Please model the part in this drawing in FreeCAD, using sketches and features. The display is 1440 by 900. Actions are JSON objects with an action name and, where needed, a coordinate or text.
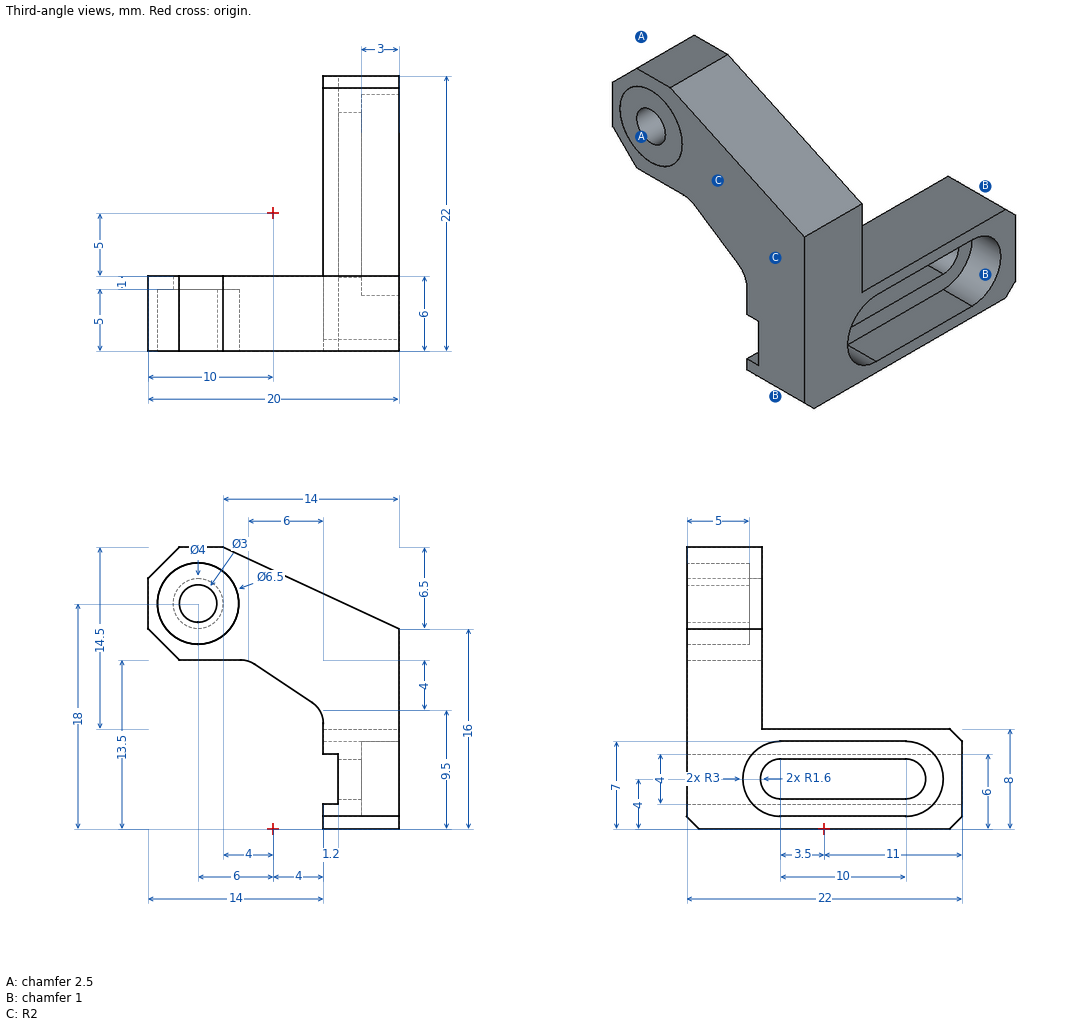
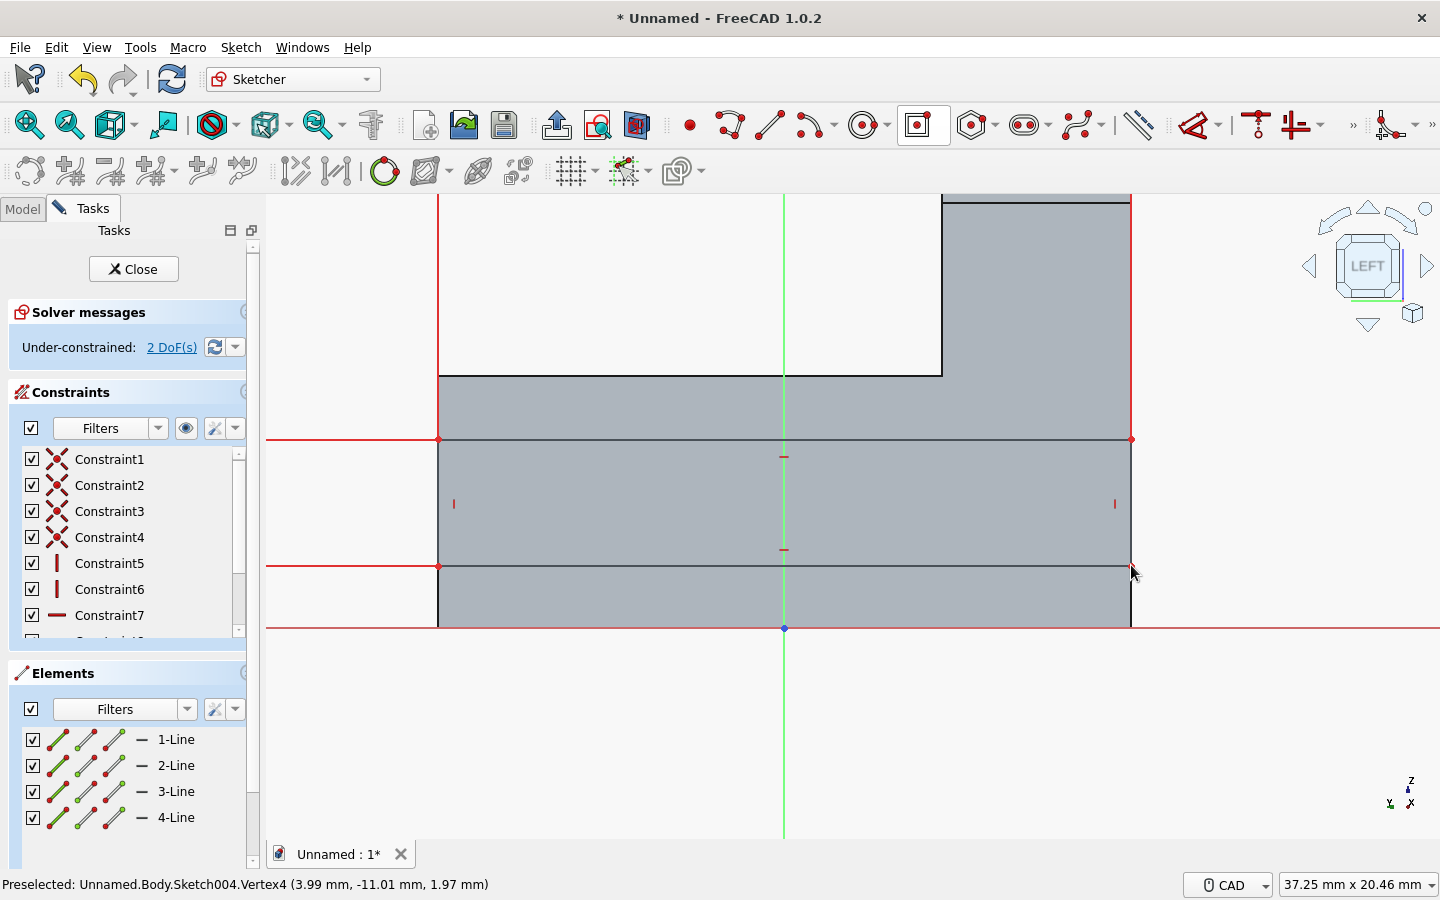
{"action": "left_click", "coordinate": [1194, 126]}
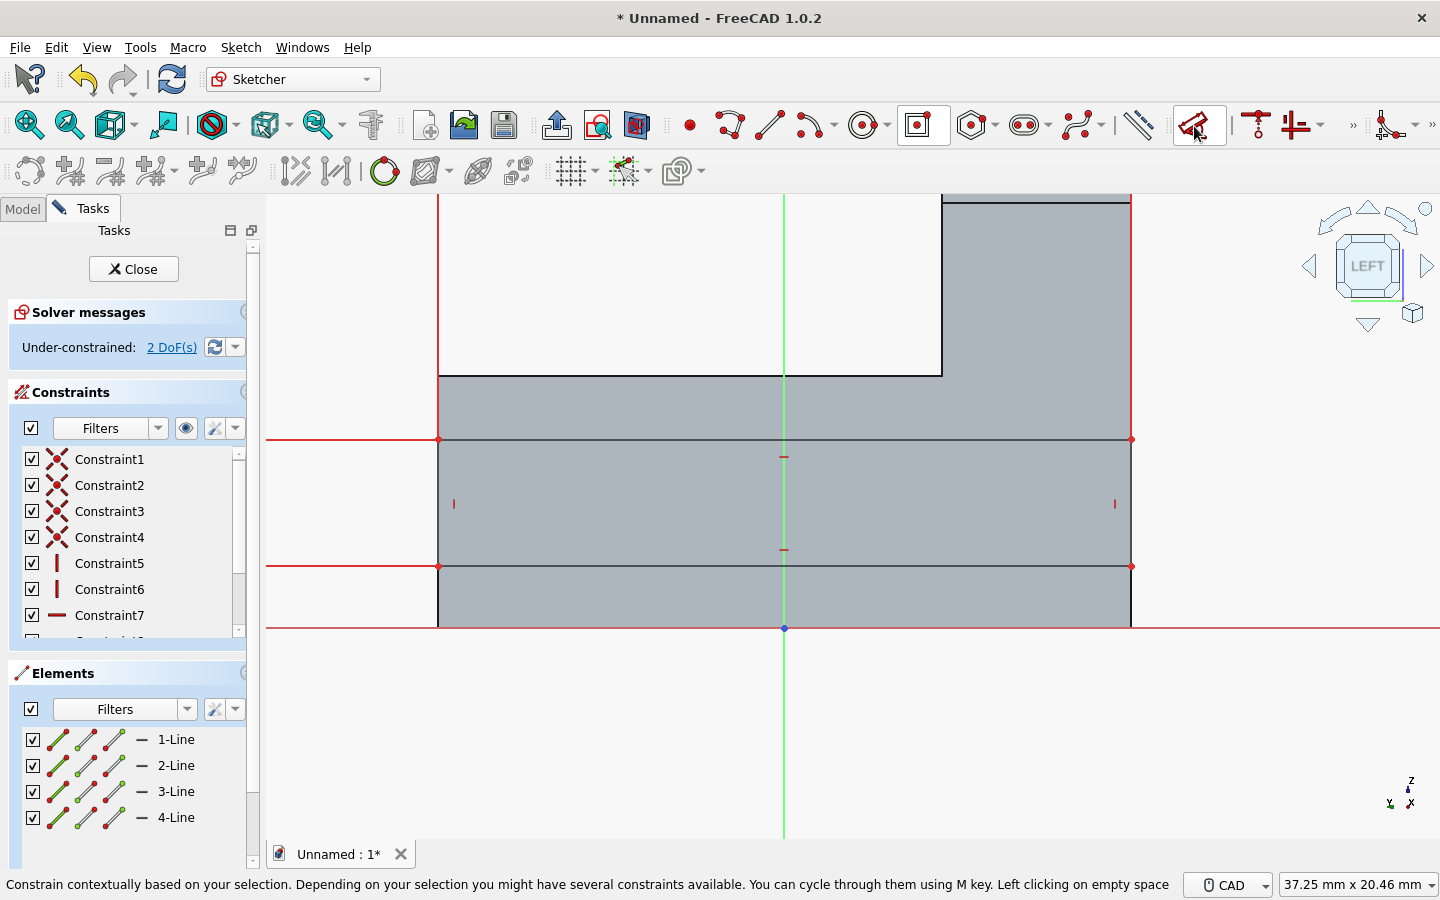
{"action": "left_click", "coordinate": [438, 440]}
{"action": "left_click", "coordinate": [404, 534]}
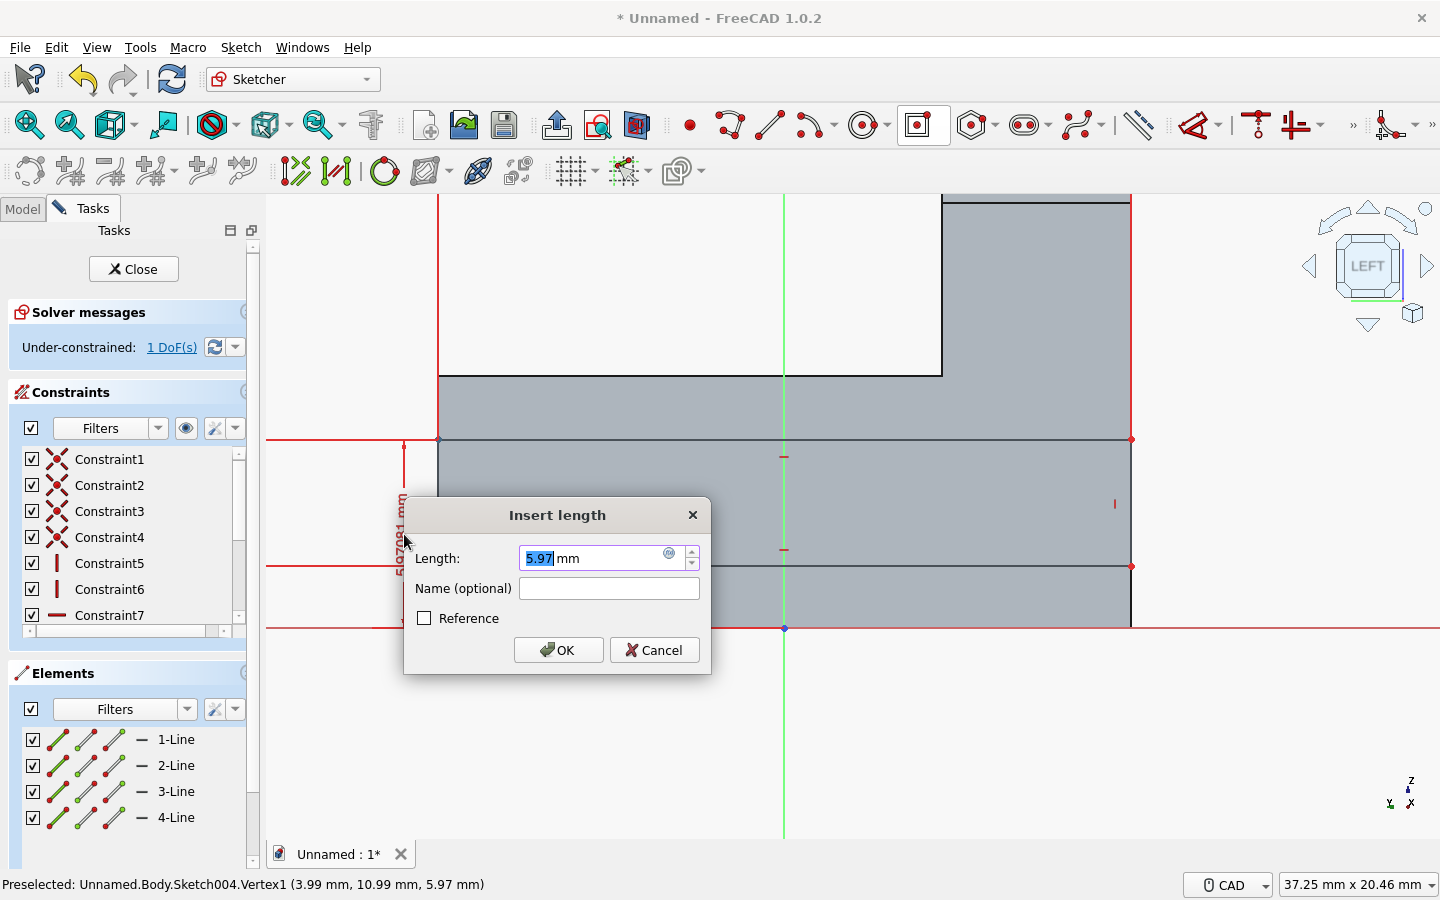
{"action": "type", "text": "6"}
{"action": "key", "text": "Return"}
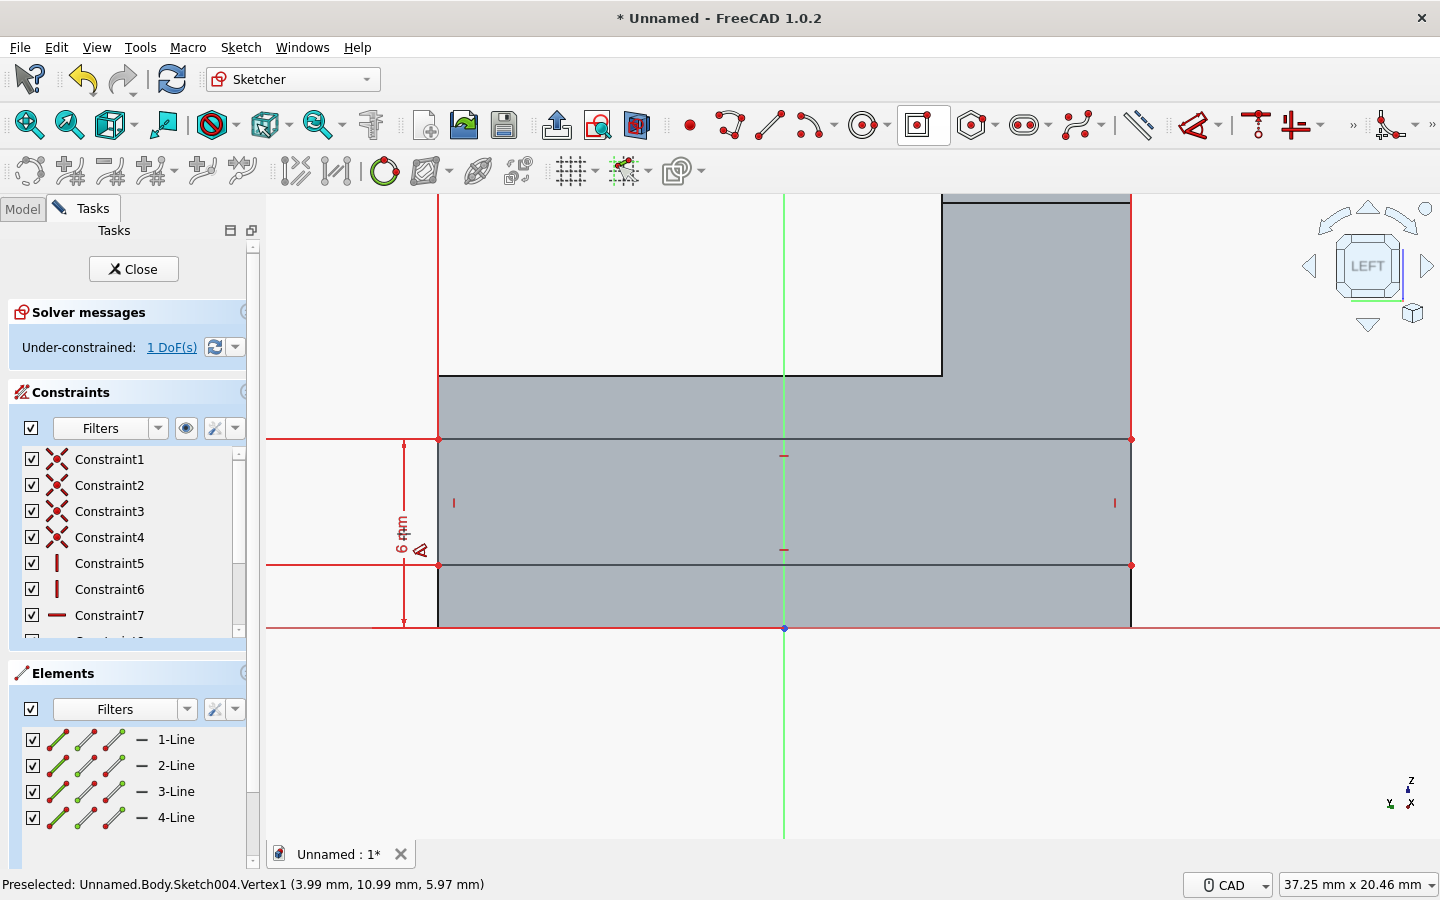
{"action": "left_click", "coordinate": [438, 439]}
{"action": "left_click", "coordinate": [611, 662]}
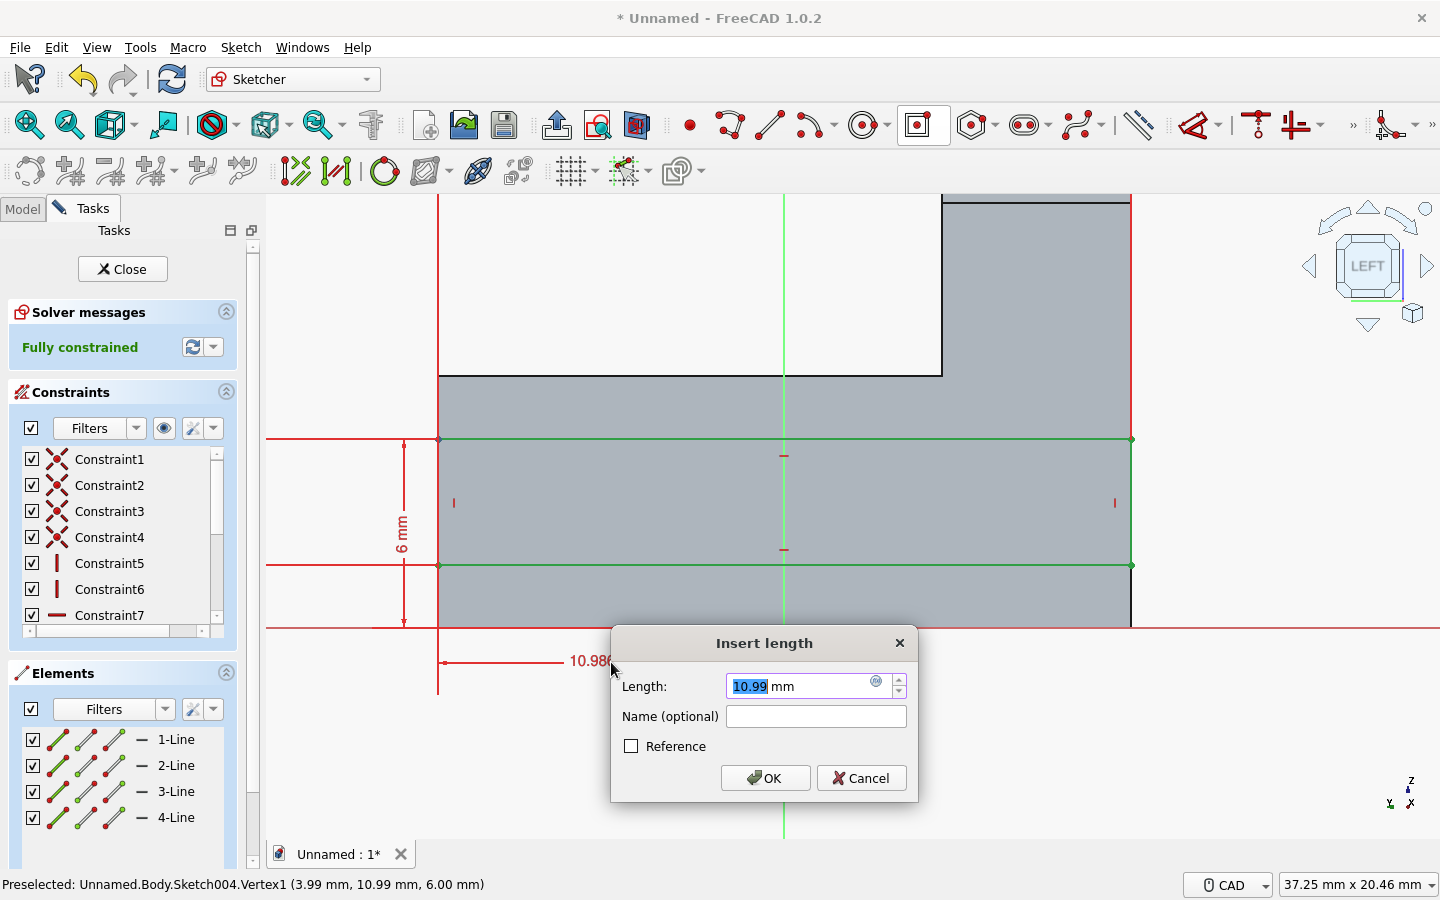
{"action": "type", "text": "11"}
{"action": "key", "text": "Return"}
{"action": "key", "text": "Escape"}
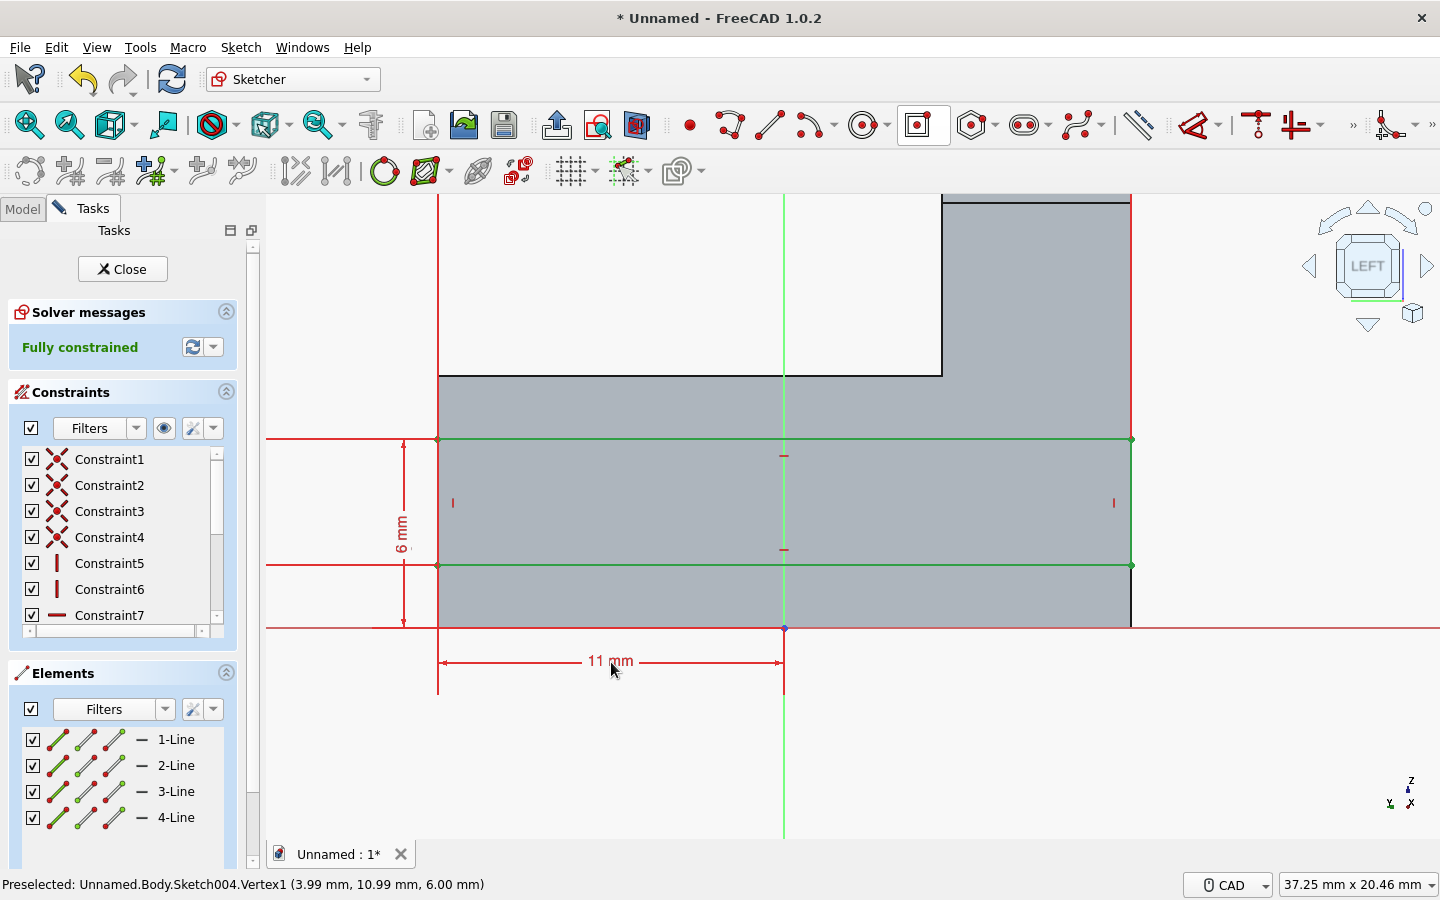
{"action": "left_click", "coordinate": [123, 269]}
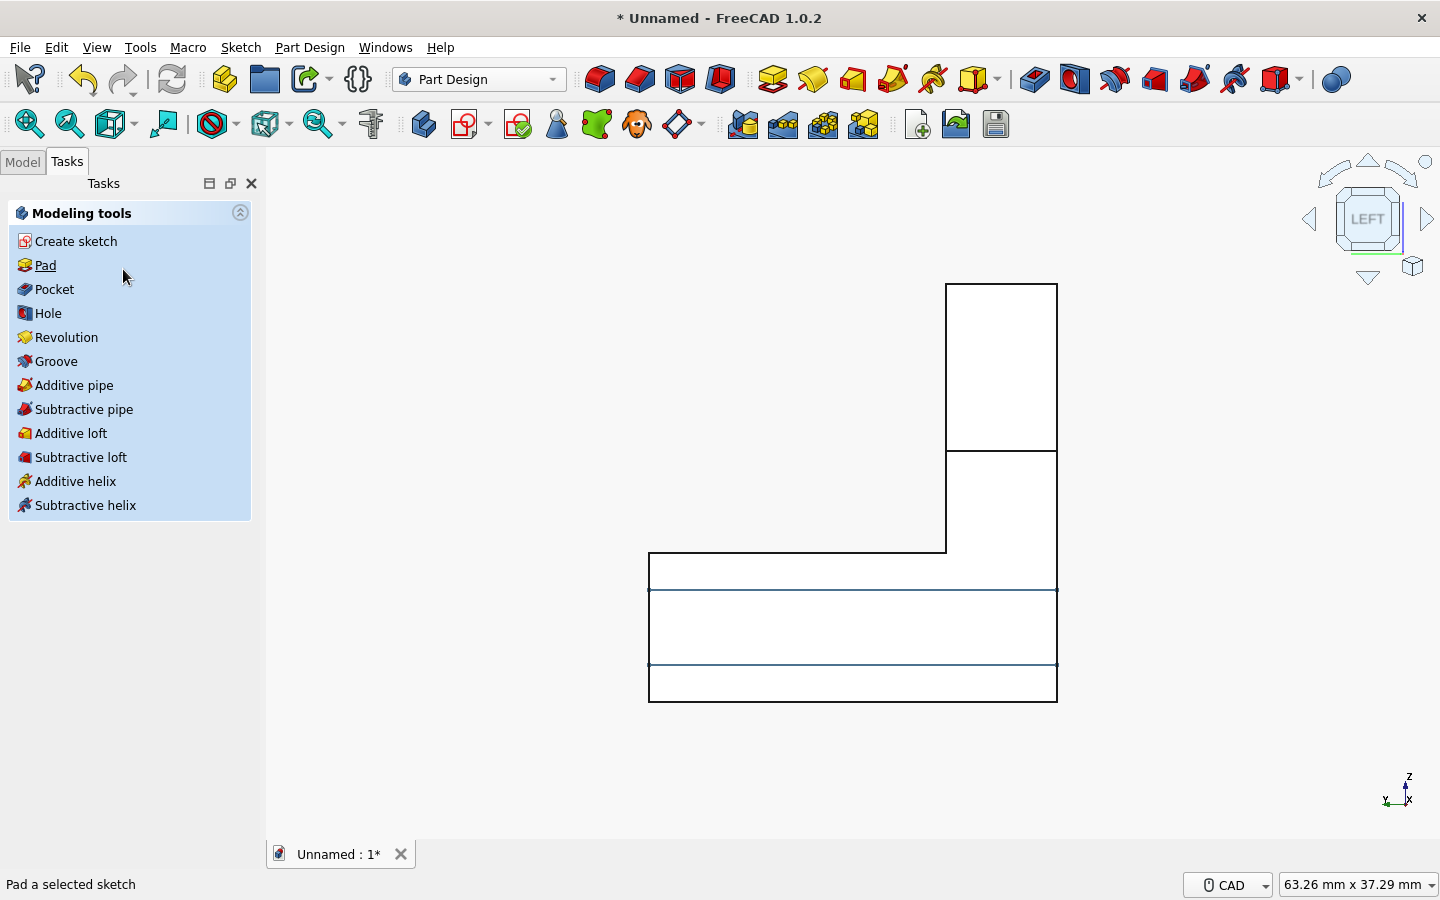
{"action": "left_click", "coordinate": [1036, 80]}